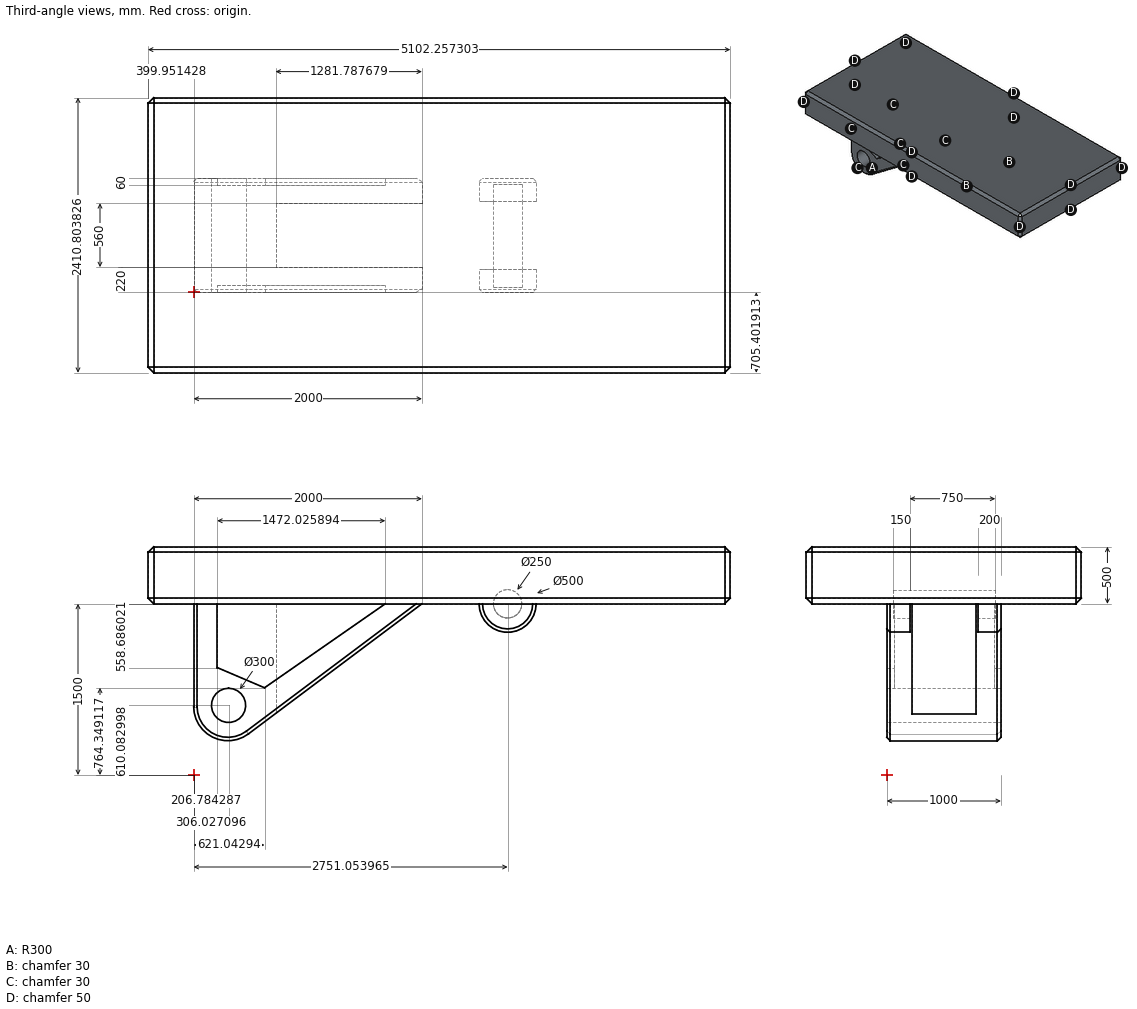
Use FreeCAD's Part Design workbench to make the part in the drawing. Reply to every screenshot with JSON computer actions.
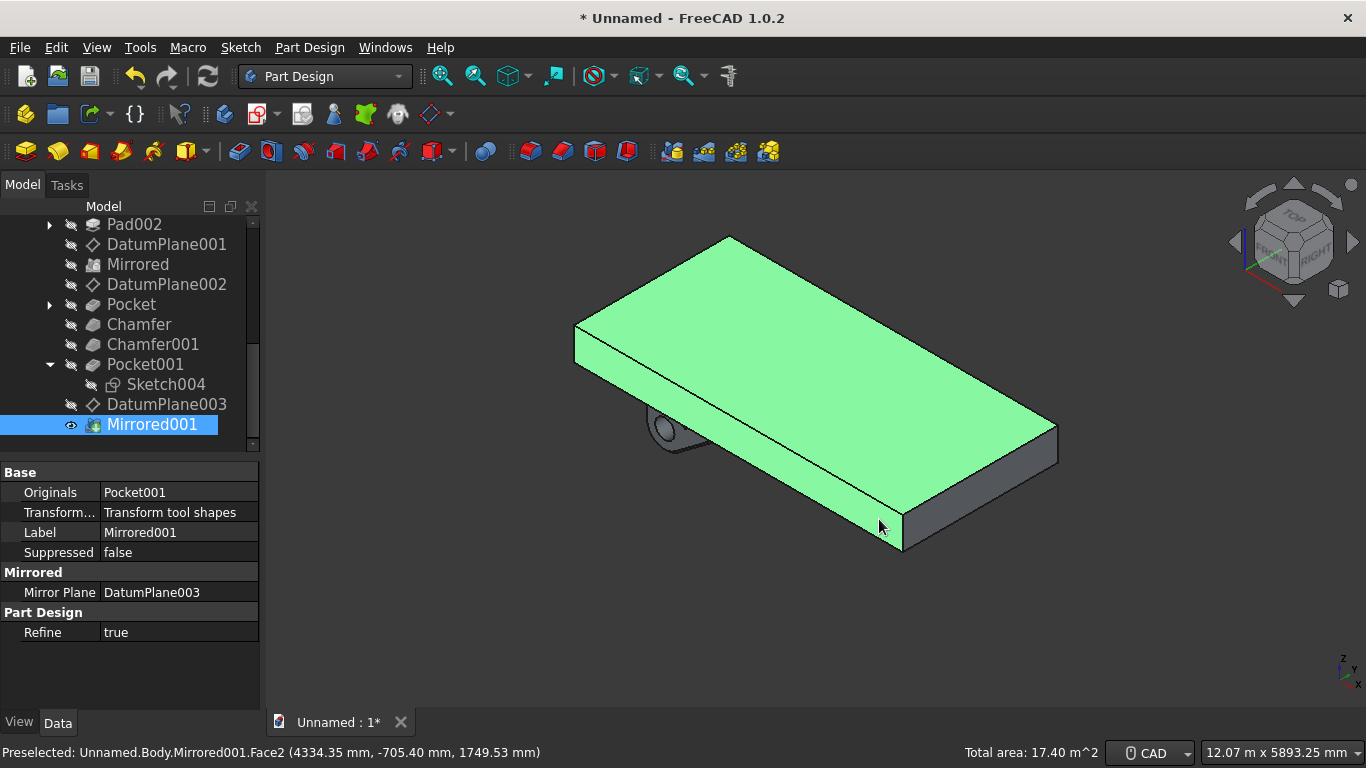
{"action": "key", "text": "2"}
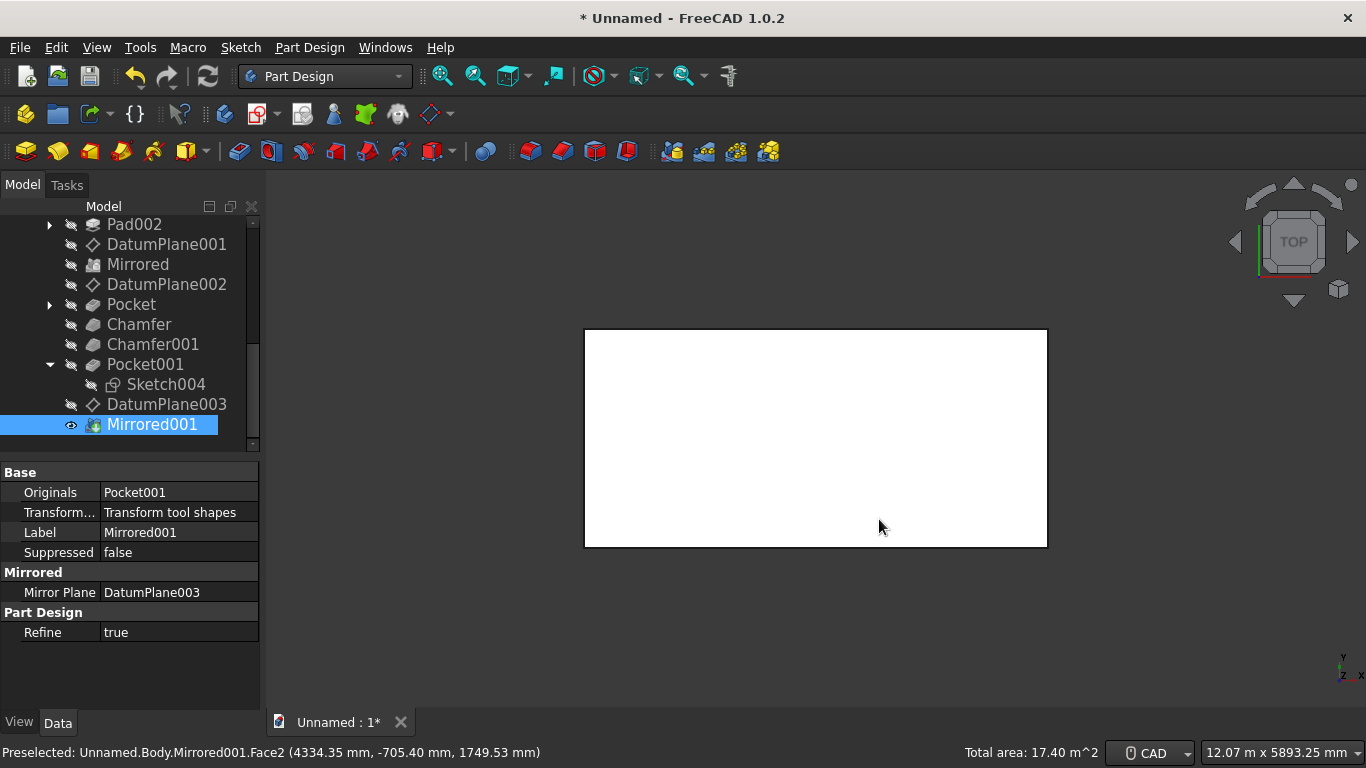
{"action": "key", "text": "v f"}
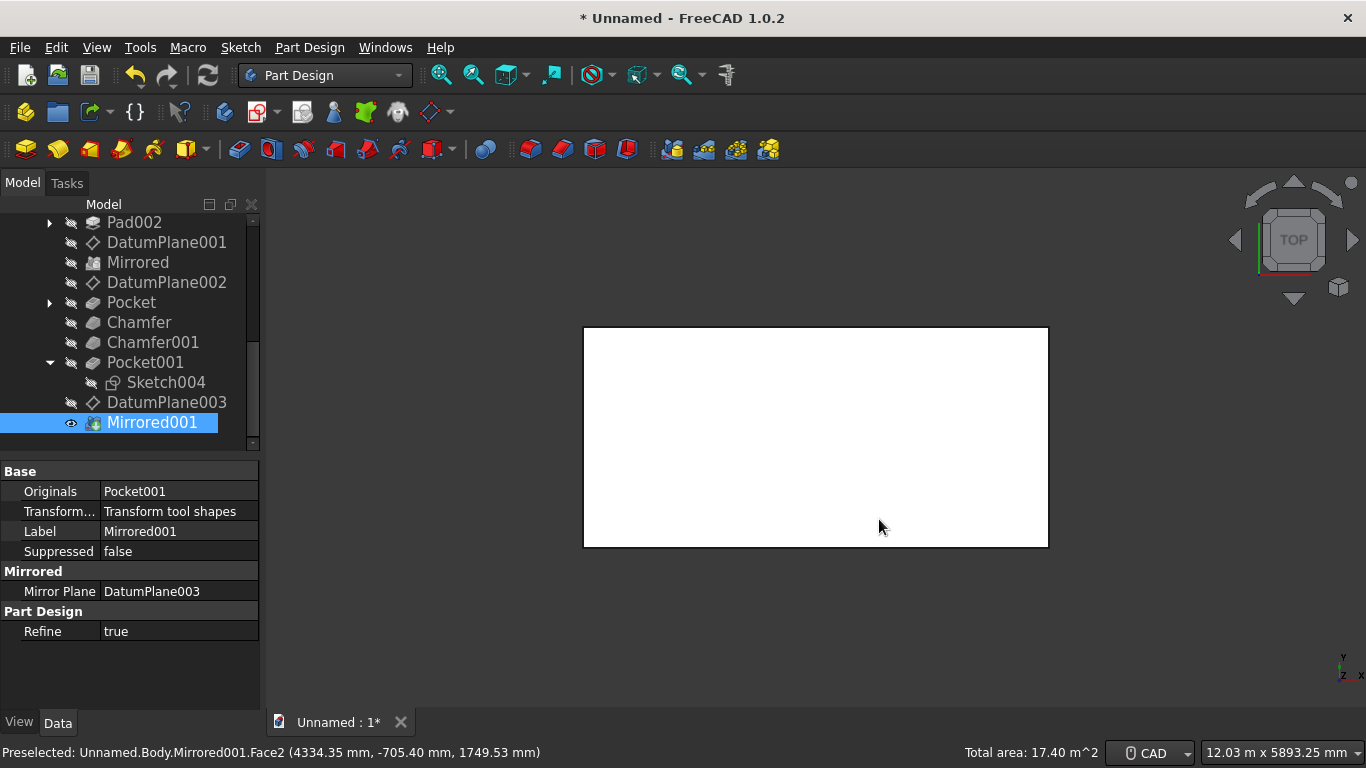
{"action": "key", "text": "1"}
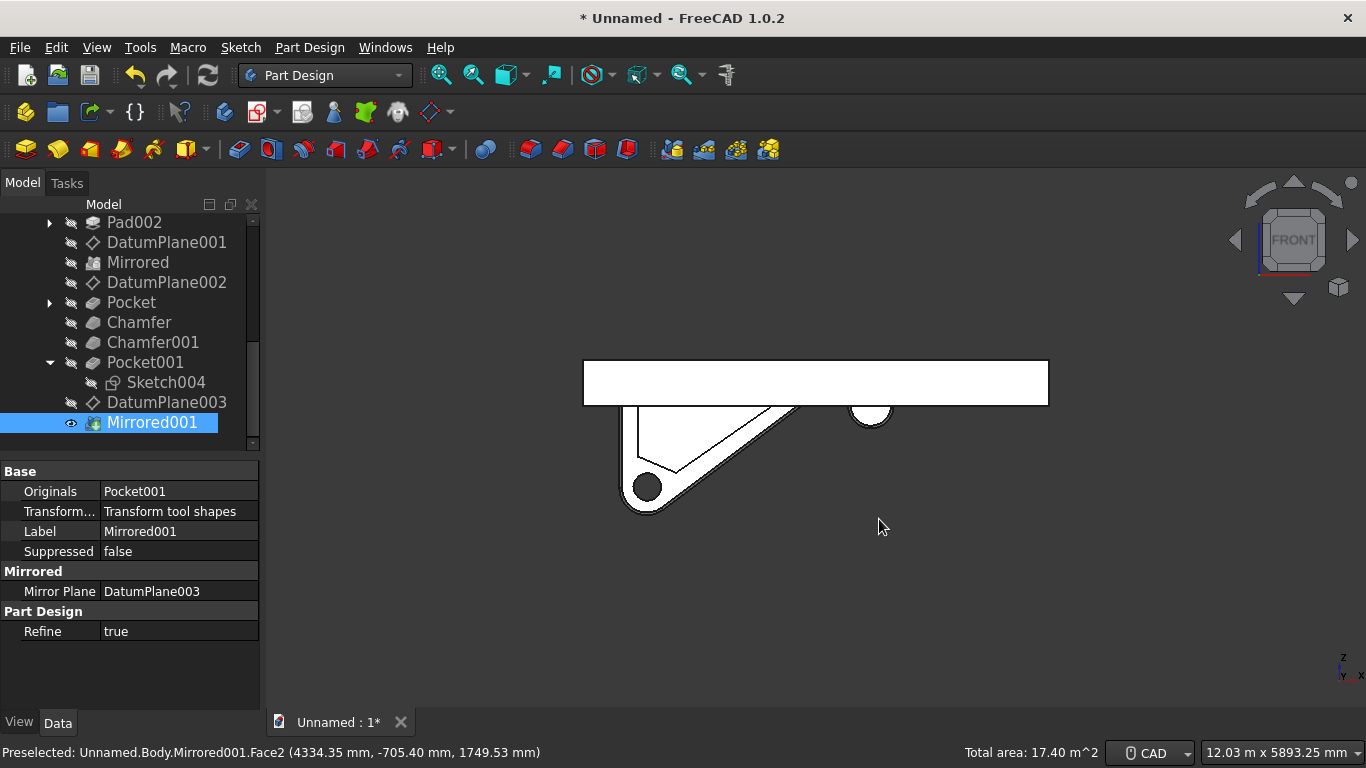
{"action": "left_click", "coordinate": [442, 76]}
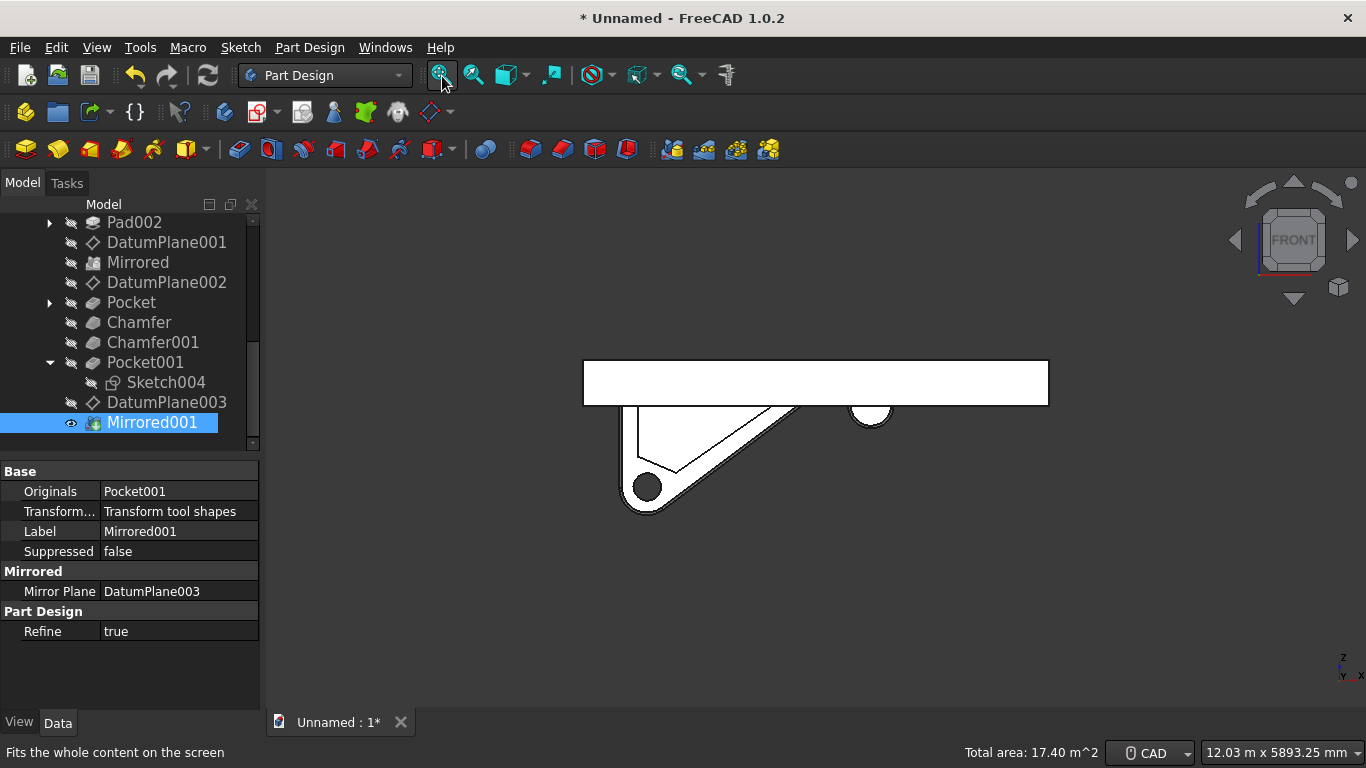
{"action": "key", "text": "3"}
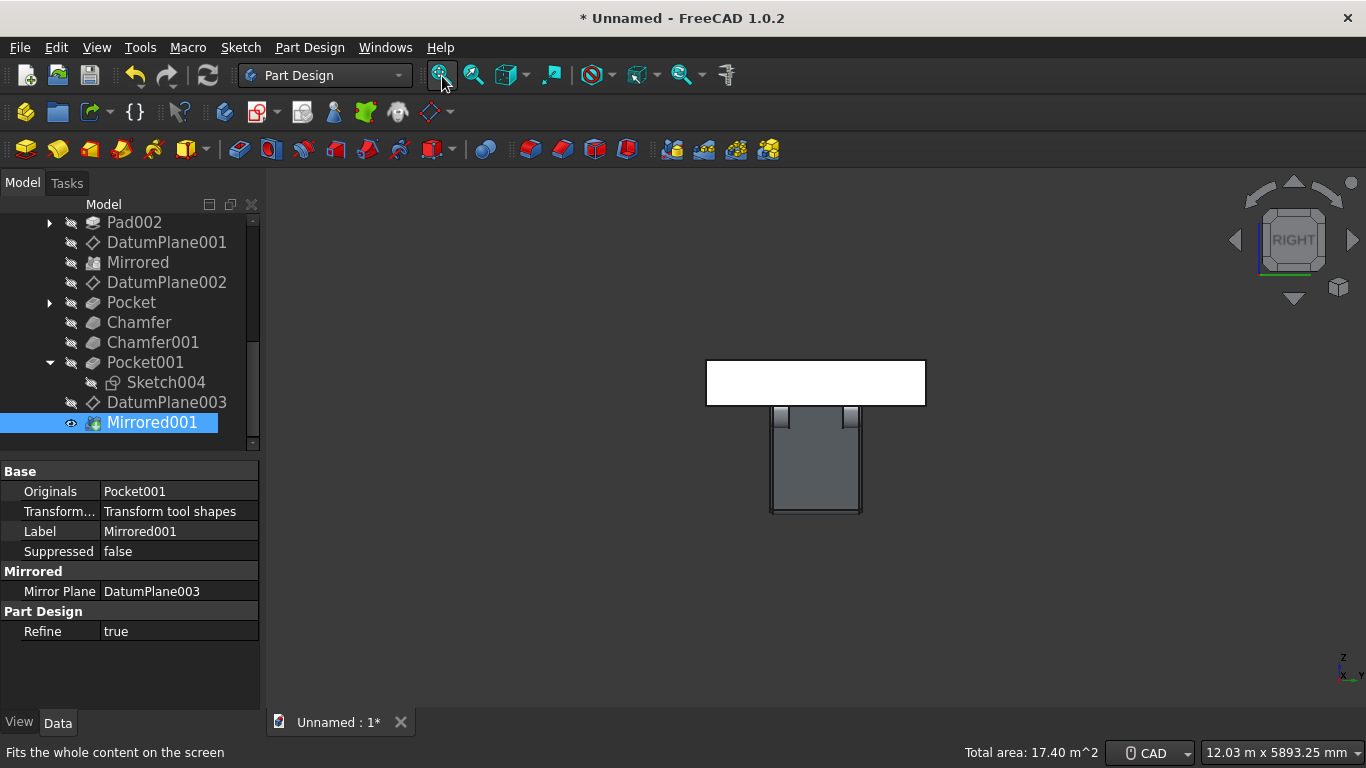
{"action": "left_click", "coordinate": [442, 76]}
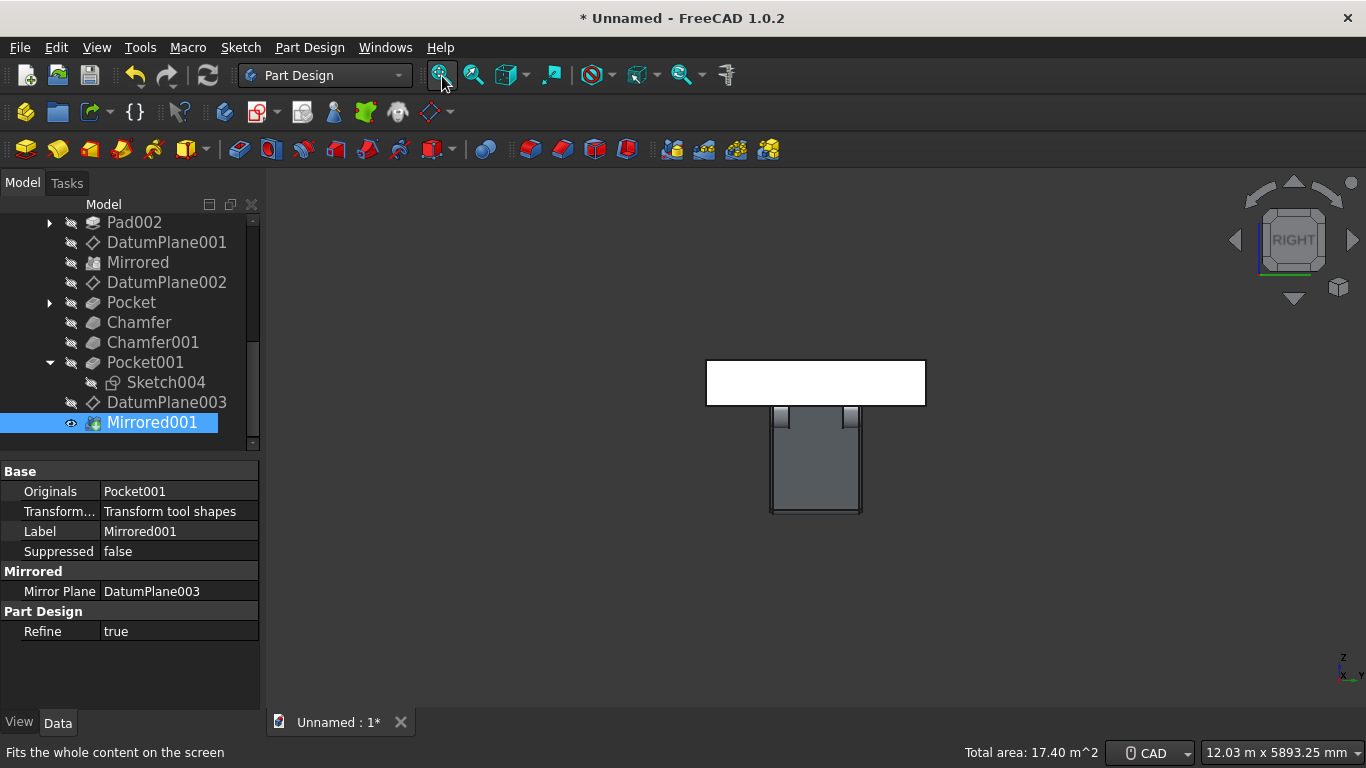
{"action": "left_click", "coordinate": [816, 405], "text": "ctrl"}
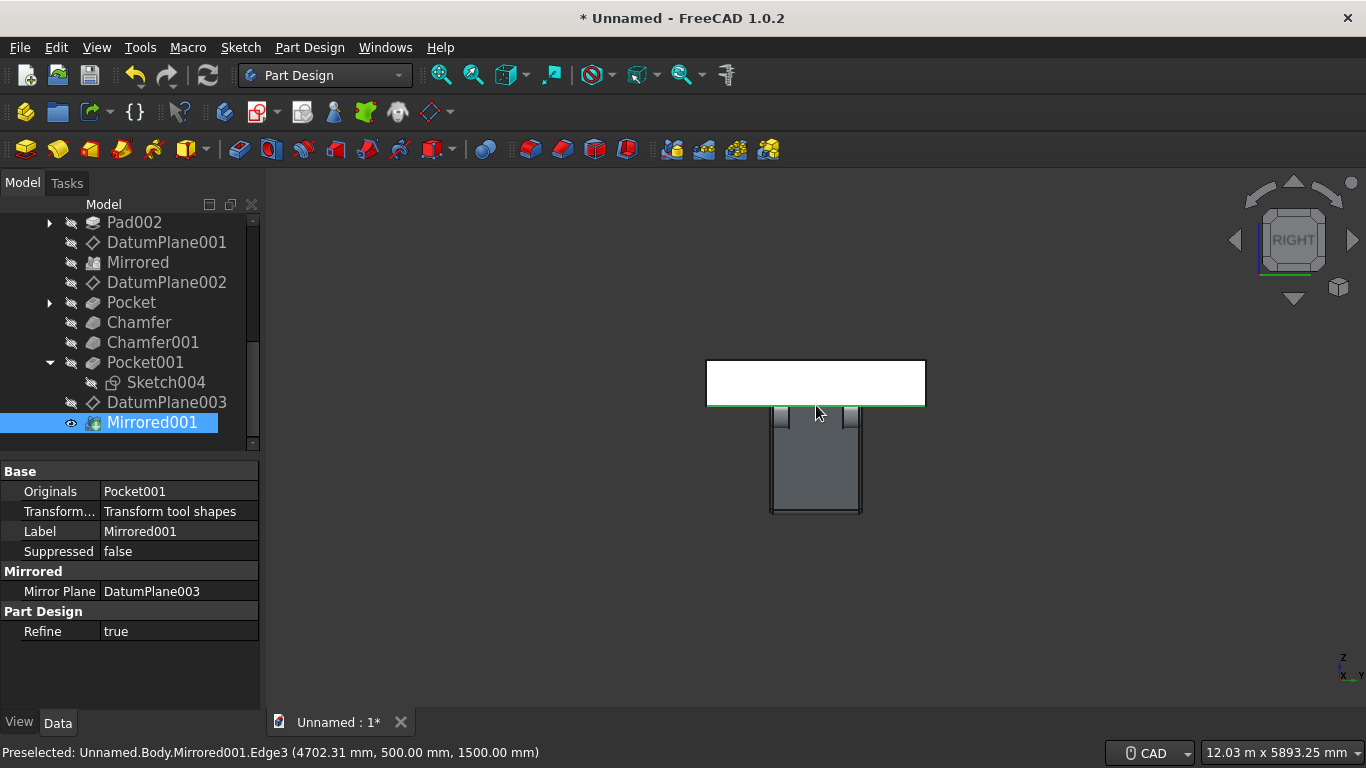
{"action": "key", "text": "5"}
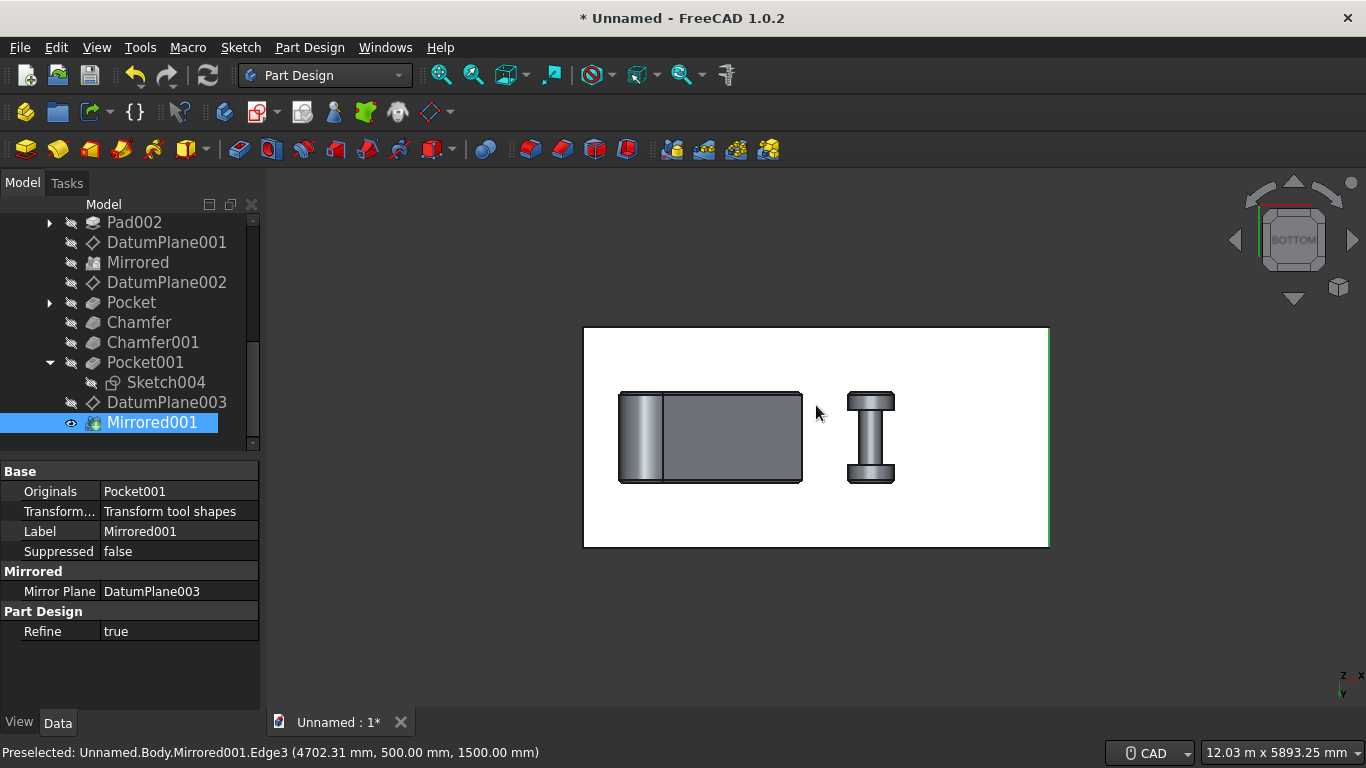
{"action": "left_click", "coordinate": [442, 76]}